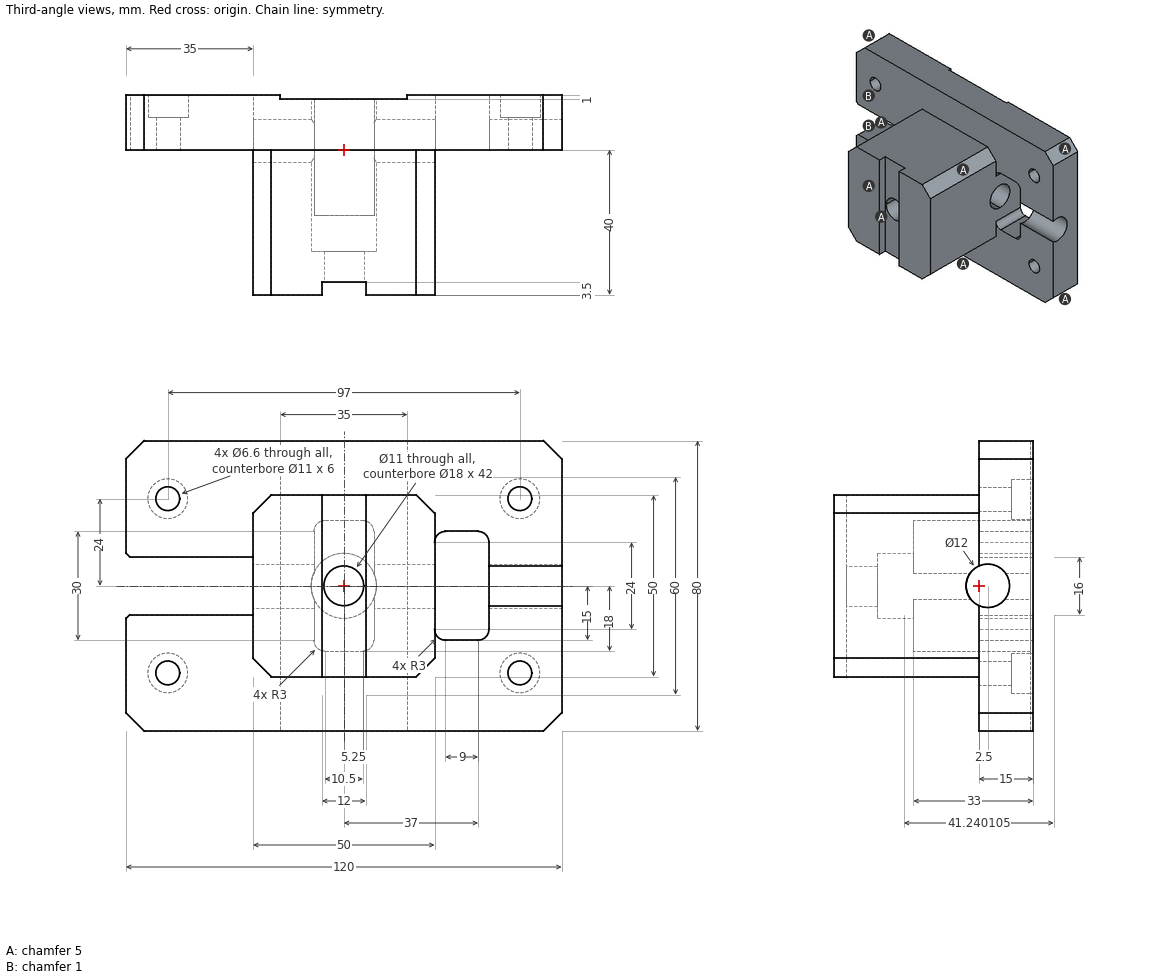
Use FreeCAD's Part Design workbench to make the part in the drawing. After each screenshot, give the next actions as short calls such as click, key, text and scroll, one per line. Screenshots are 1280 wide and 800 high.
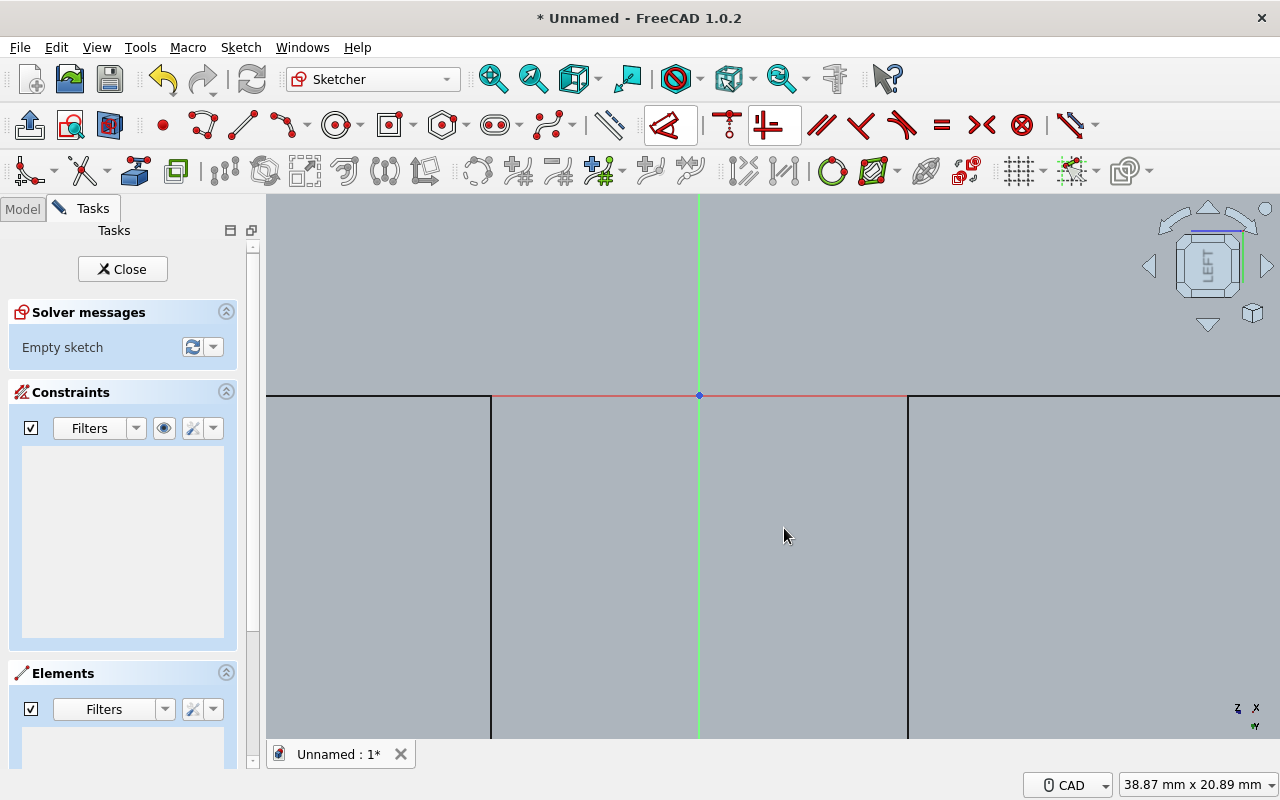
key(g)
key(c)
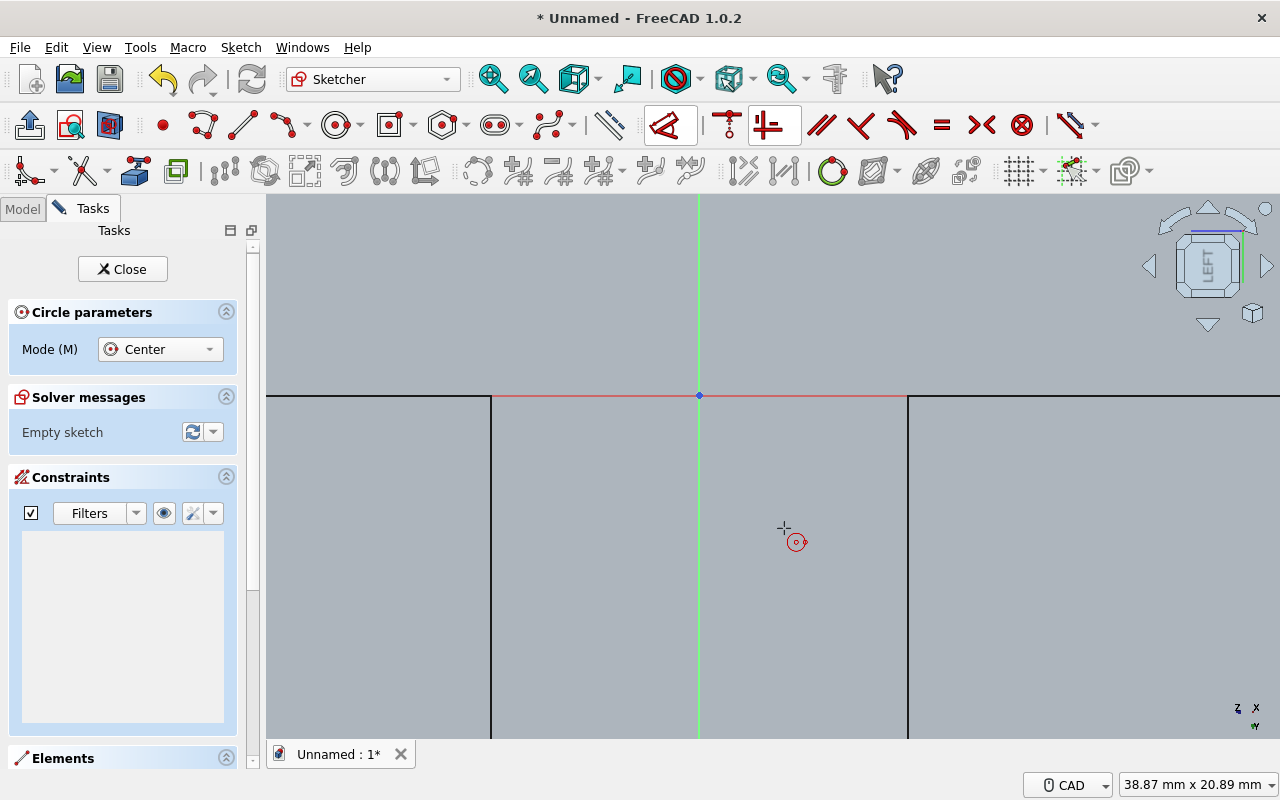
click(699, 461)
click(810, 350)
key(Escape)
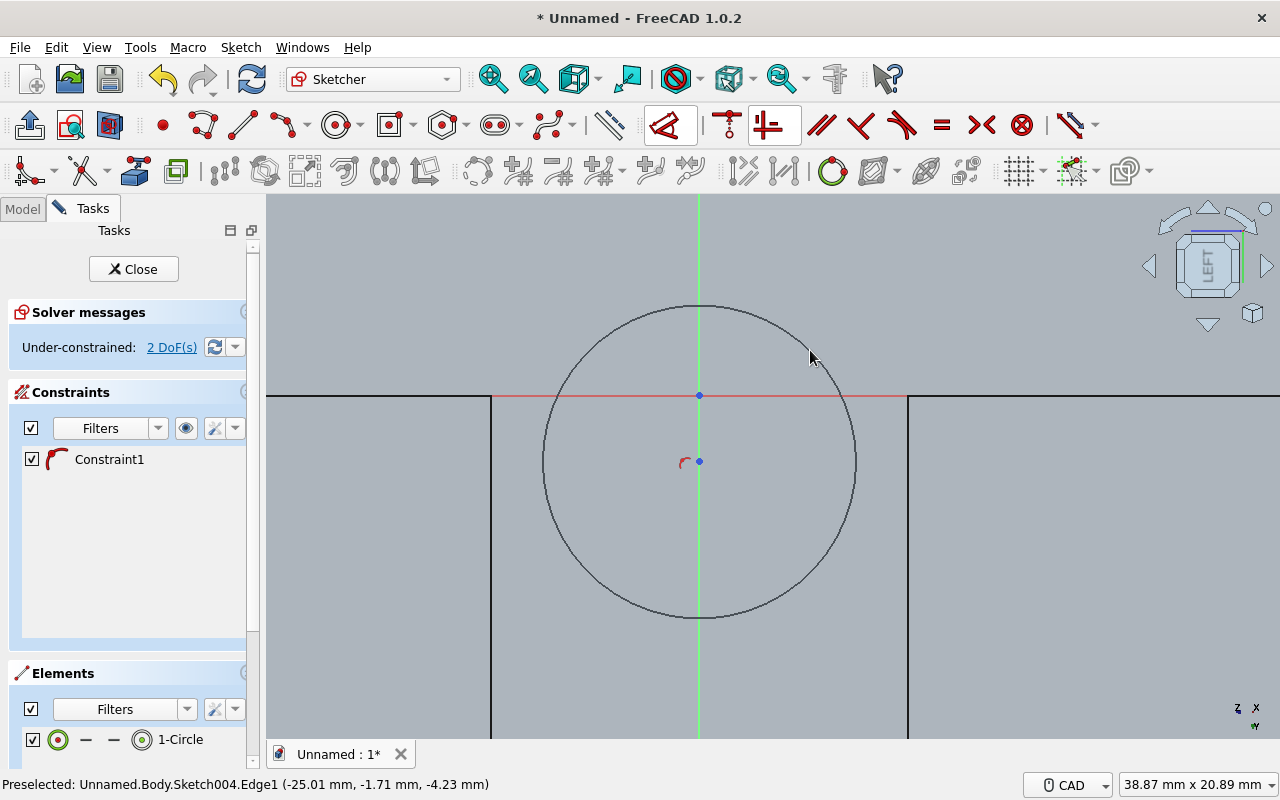
click(810, 351)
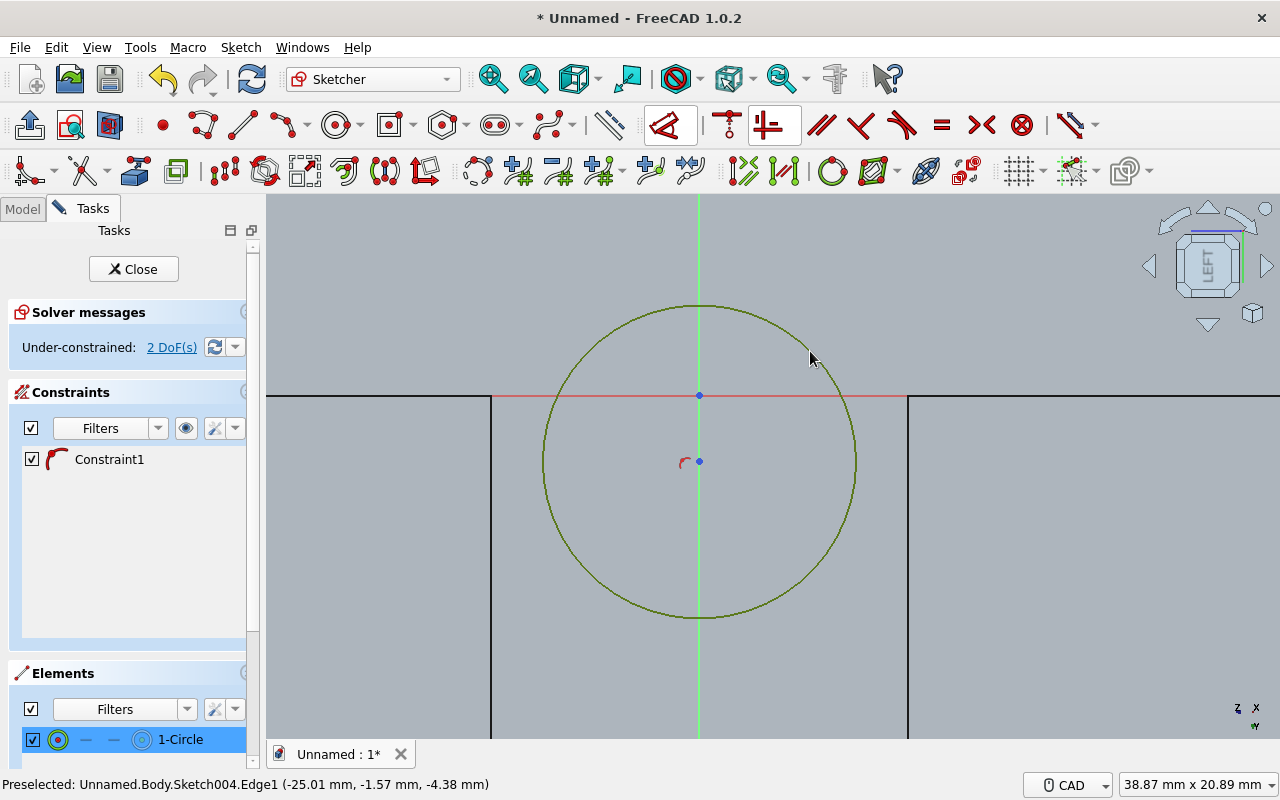
key(k)
key(o)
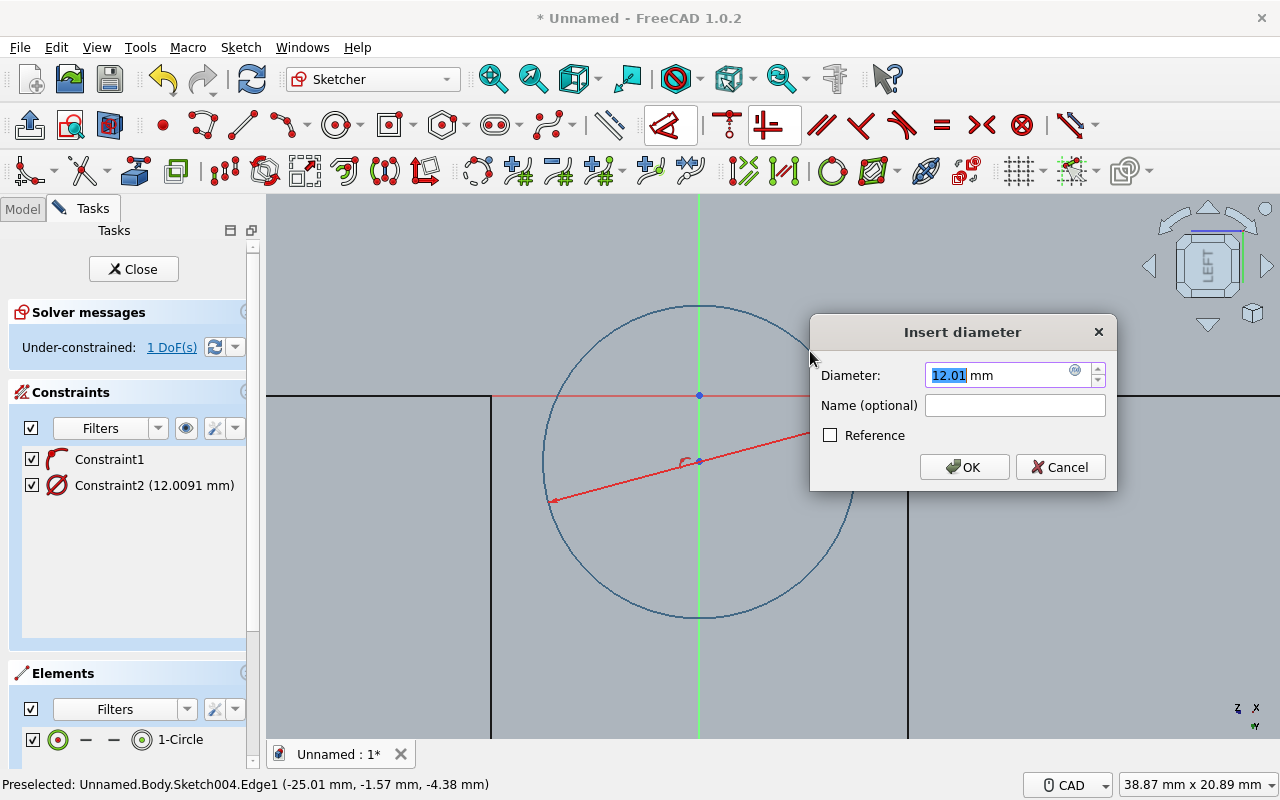
text(12)
key(Return)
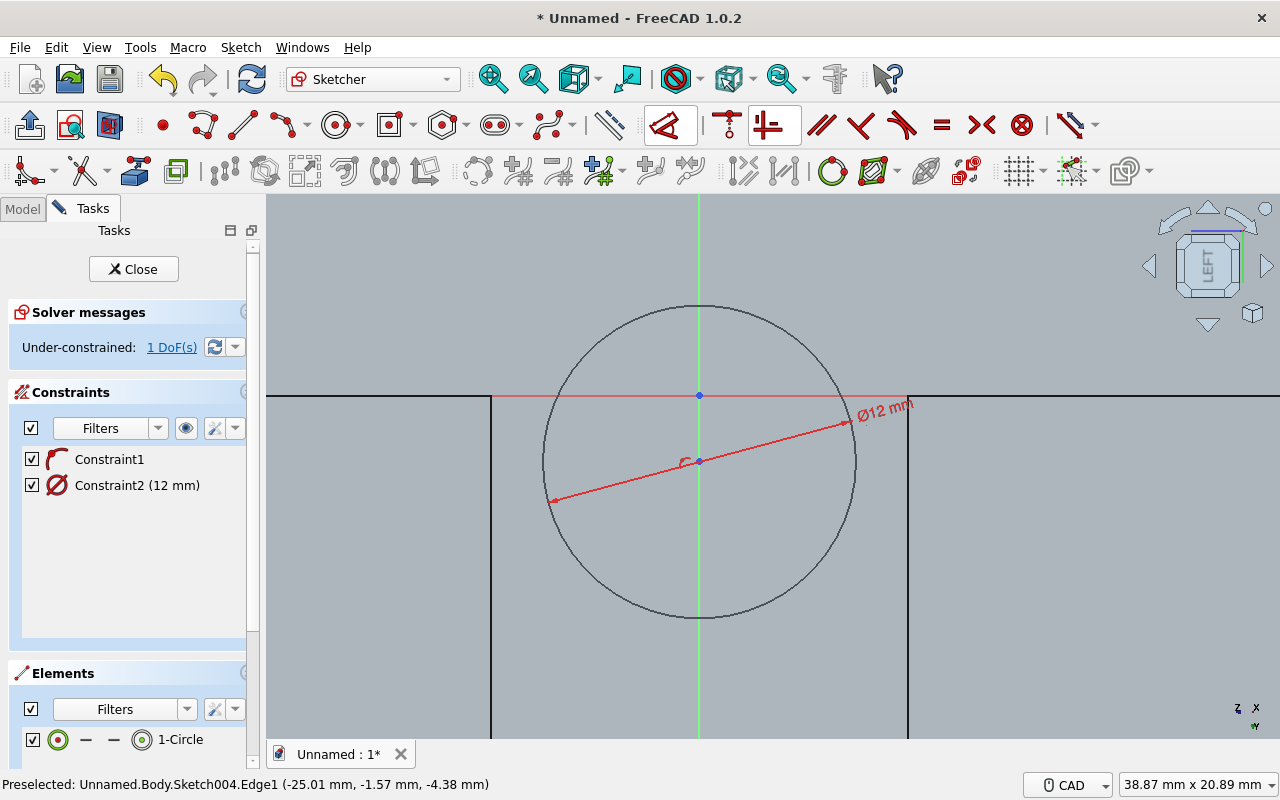
click(699, 462)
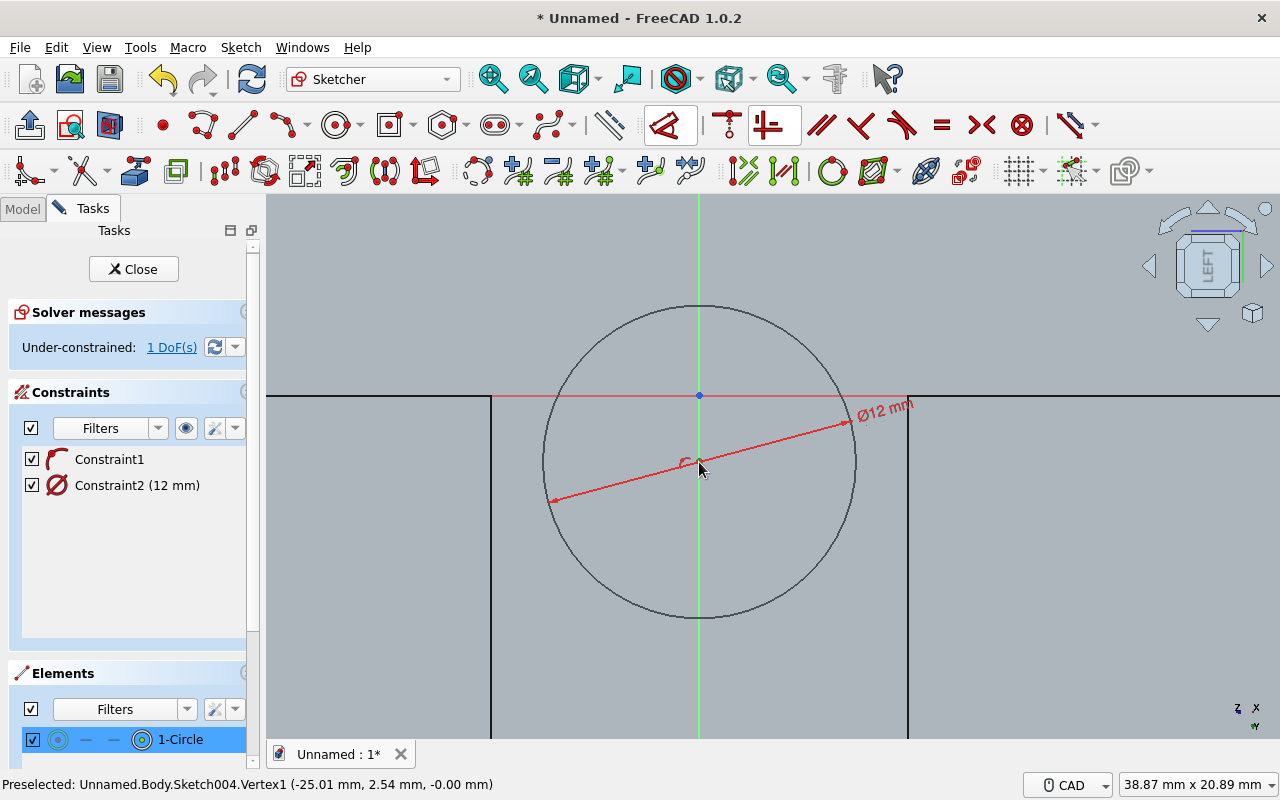
key(i)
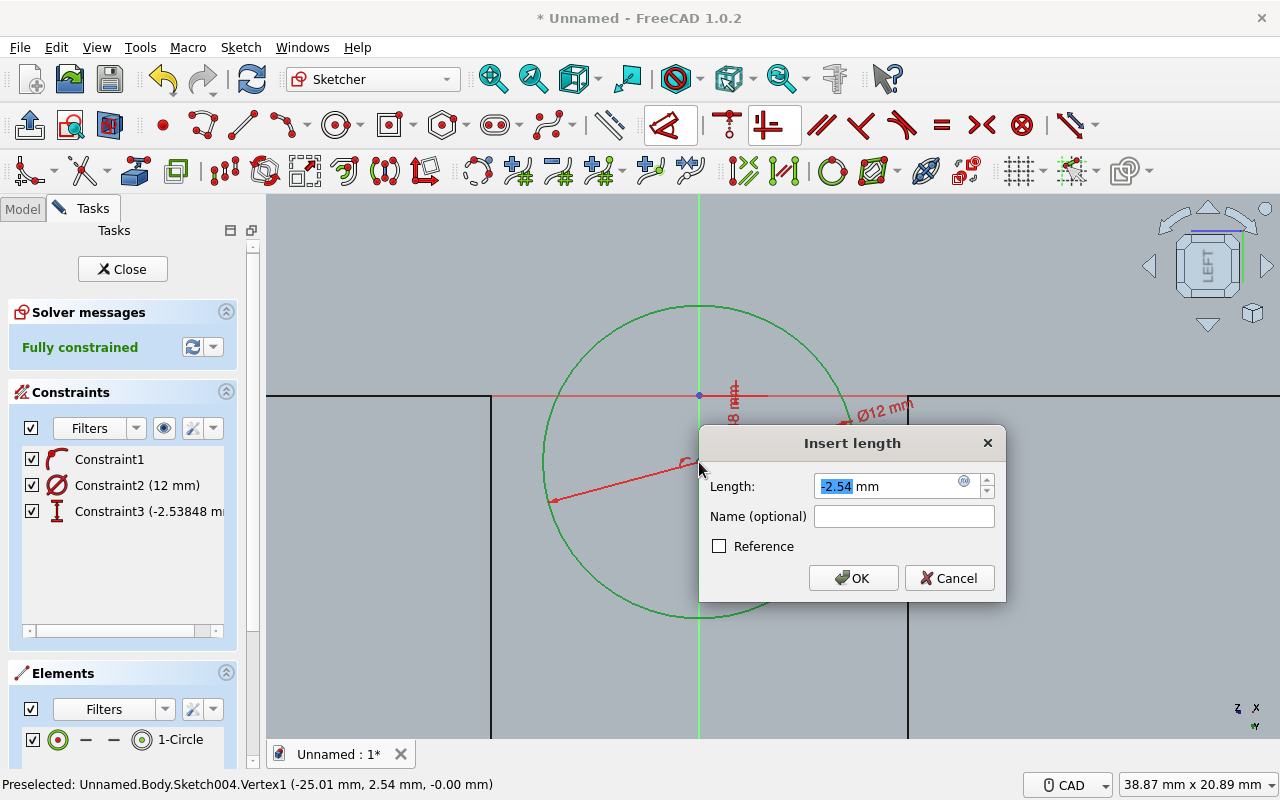
text(-2.5)
key(Return)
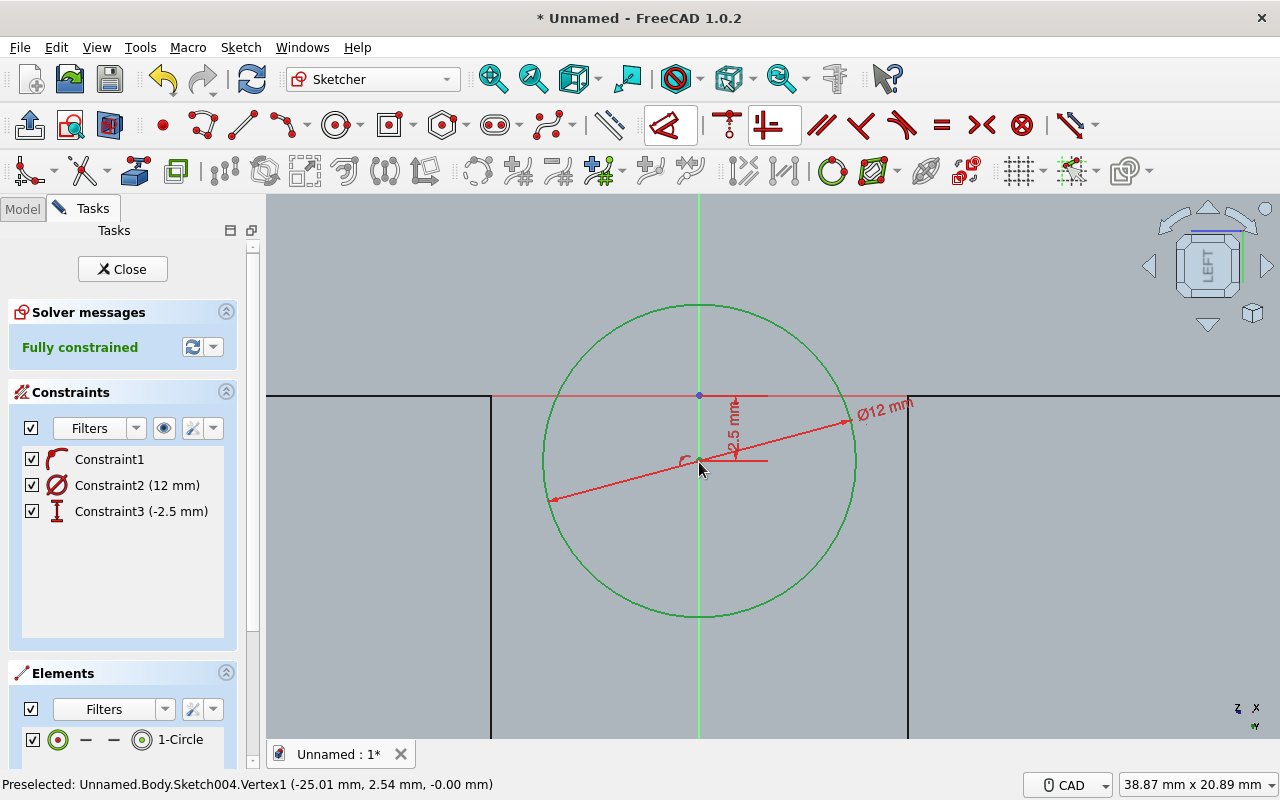
click(123, 269)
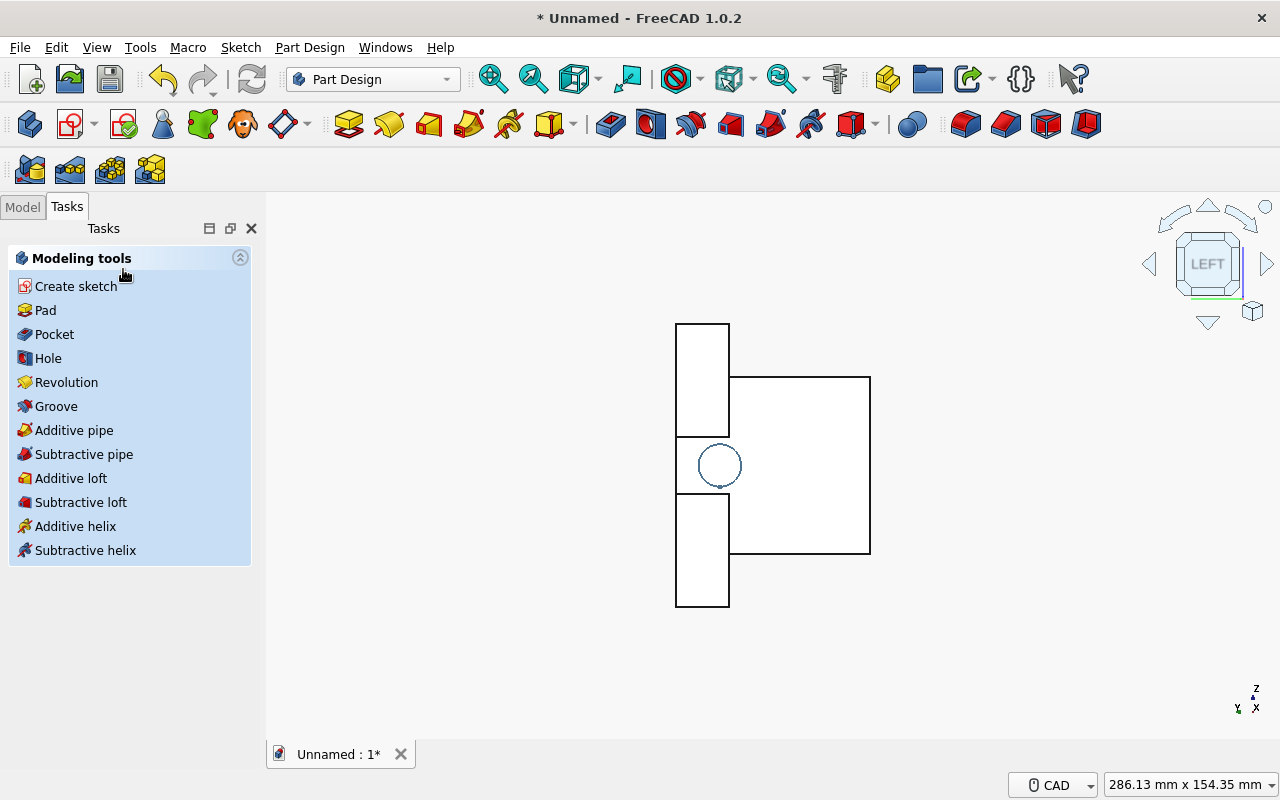
click(612, 124)